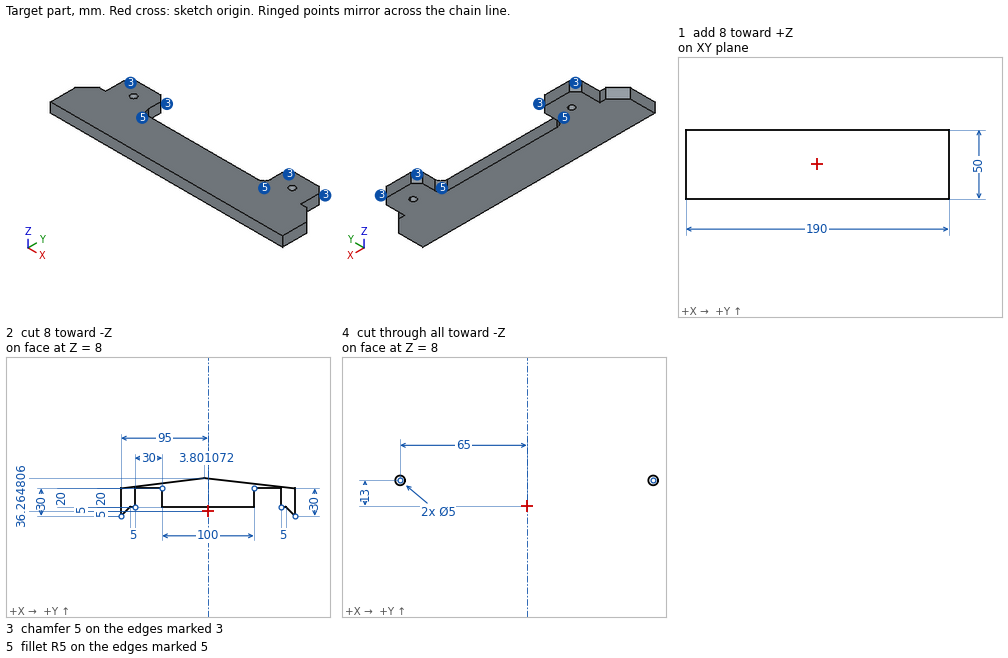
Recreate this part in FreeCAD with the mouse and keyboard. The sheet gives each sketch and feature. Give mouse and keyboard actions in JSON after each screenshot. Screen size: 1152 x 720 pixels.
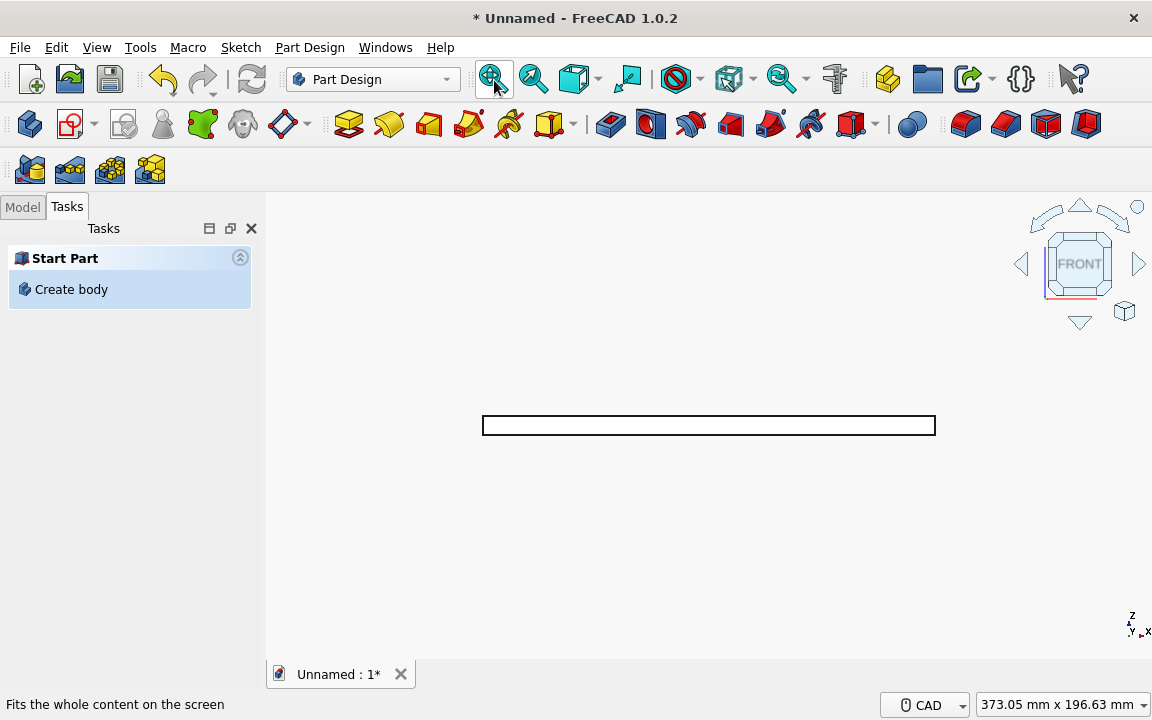
{"action": "key", "text": "3"}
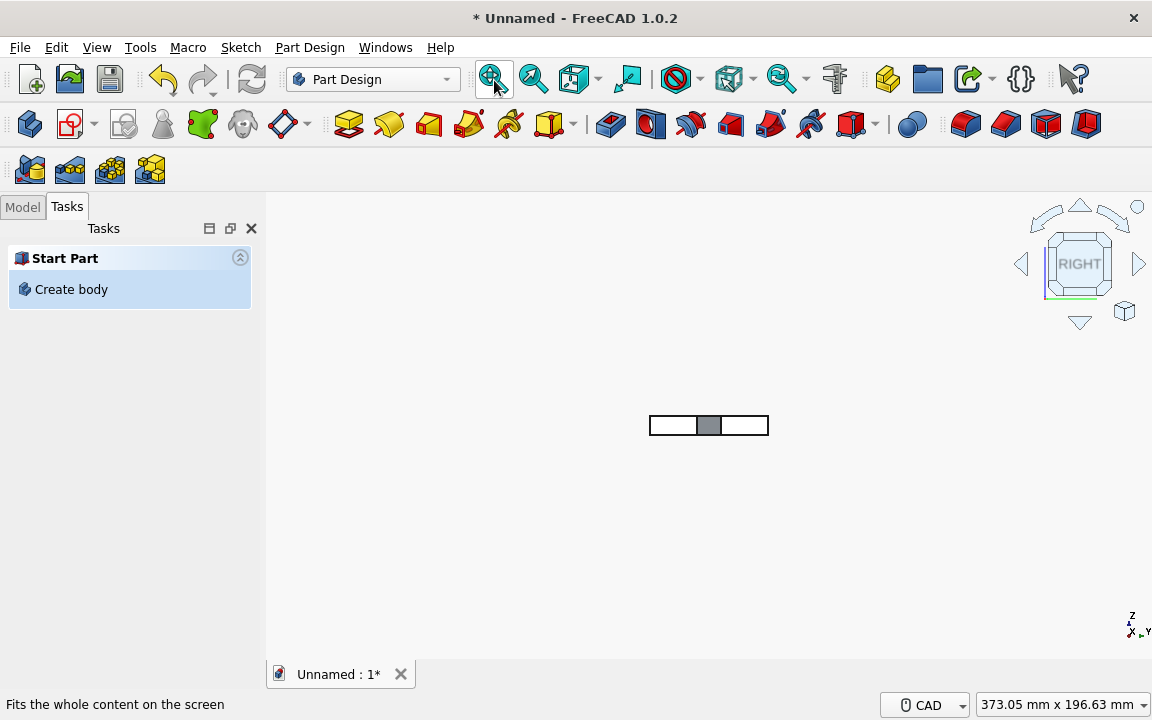
{"action": "left_click", "coordinate": [494, 80]}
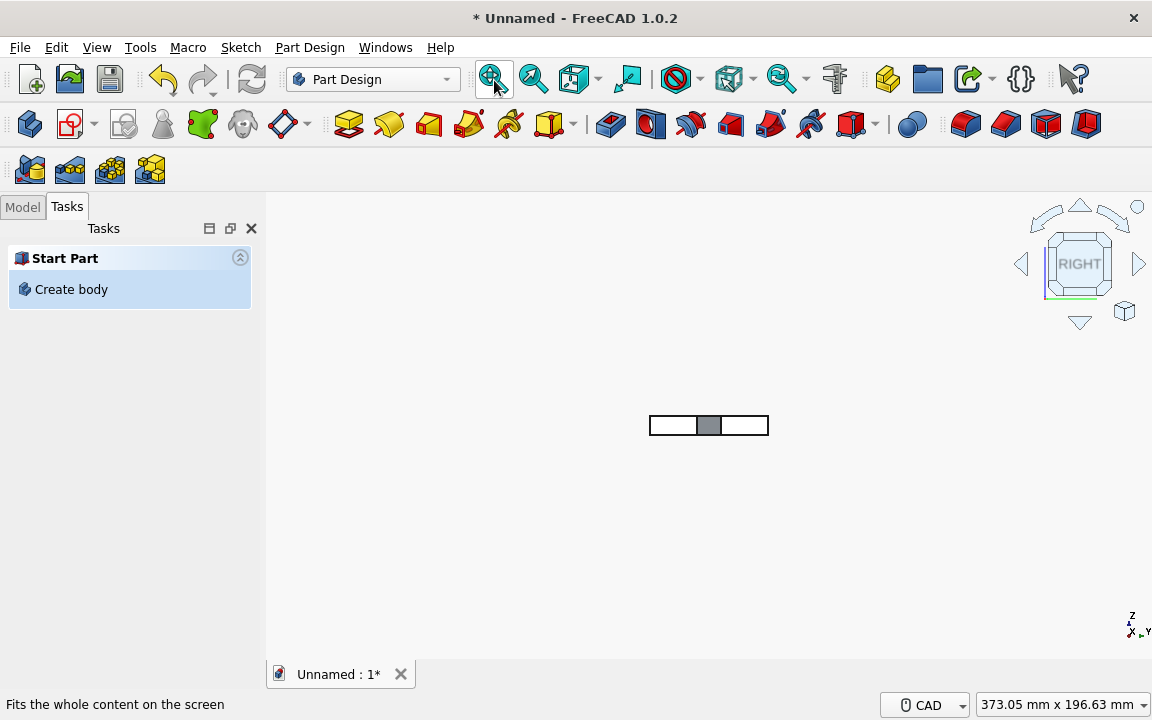
{"action": "left_click", "coordinate": [768, 424]}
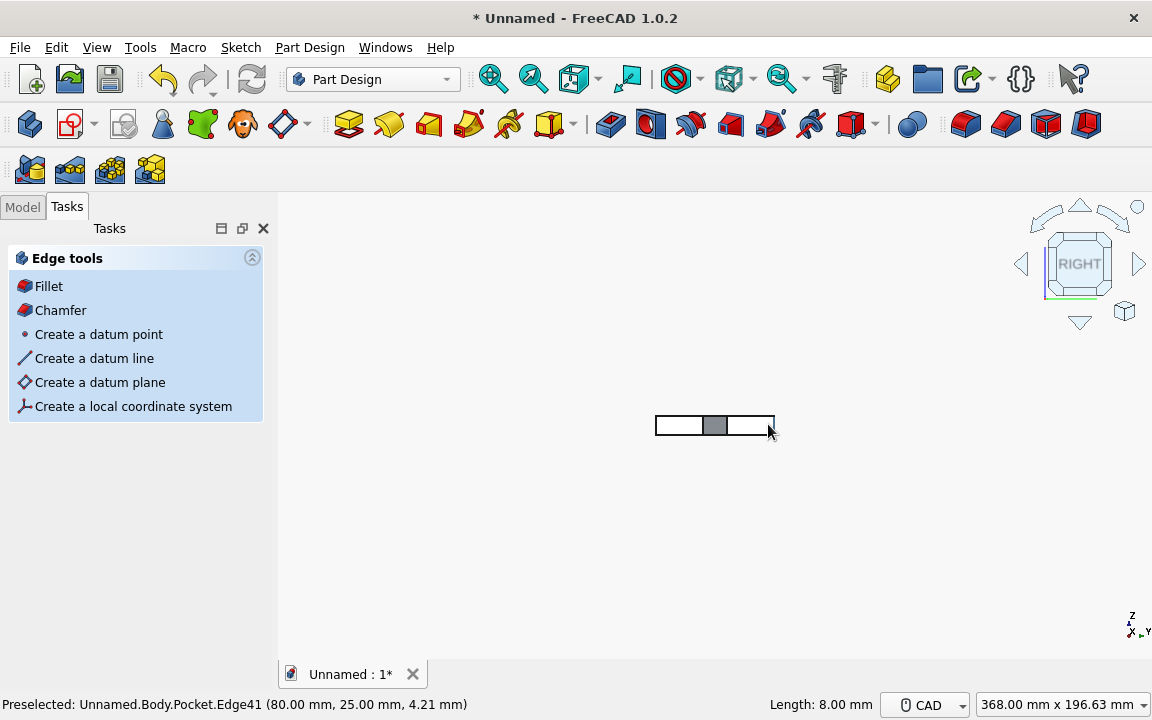
{"action": "scroll", "coordinate": [774, 424], "scroll_direction": "up", "scroll_amount": 4}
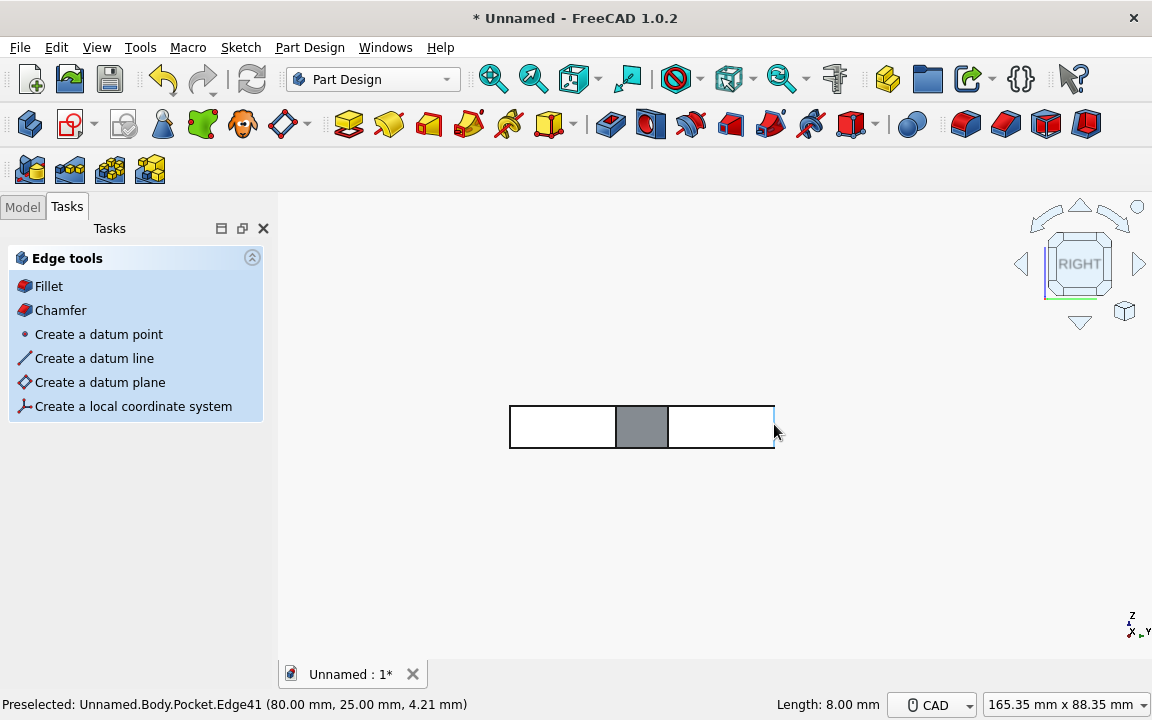
{"action": "key", "text": "v f"}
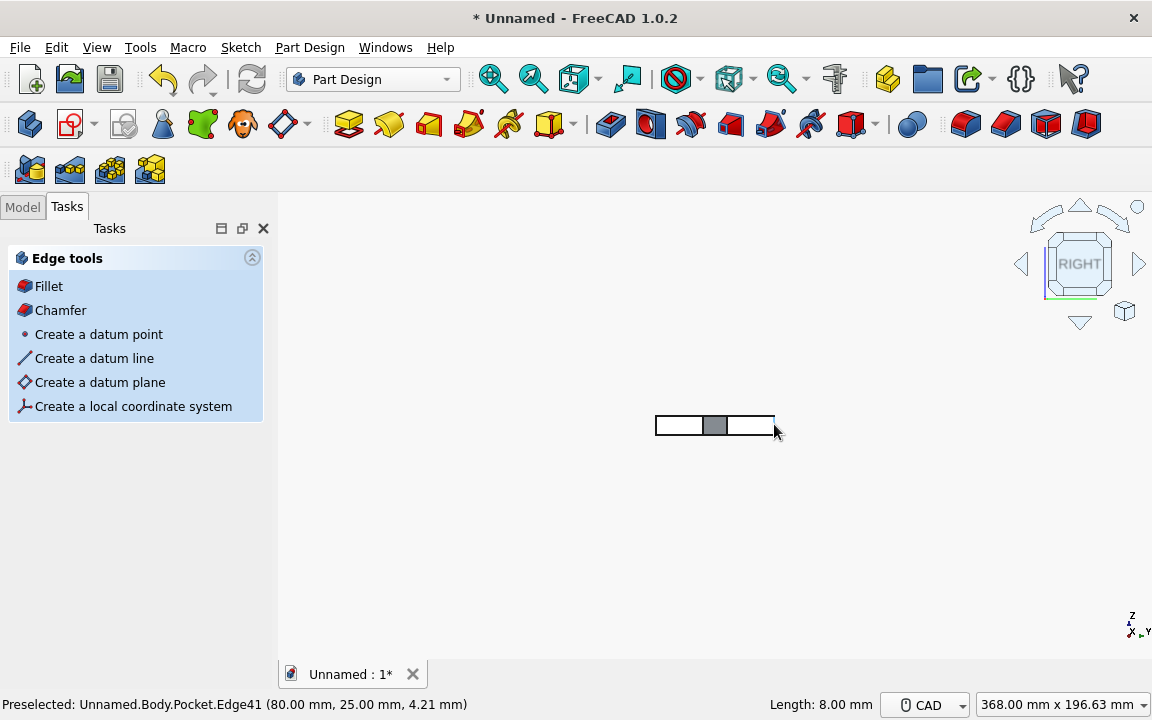
{"action": "key", "text": "5"}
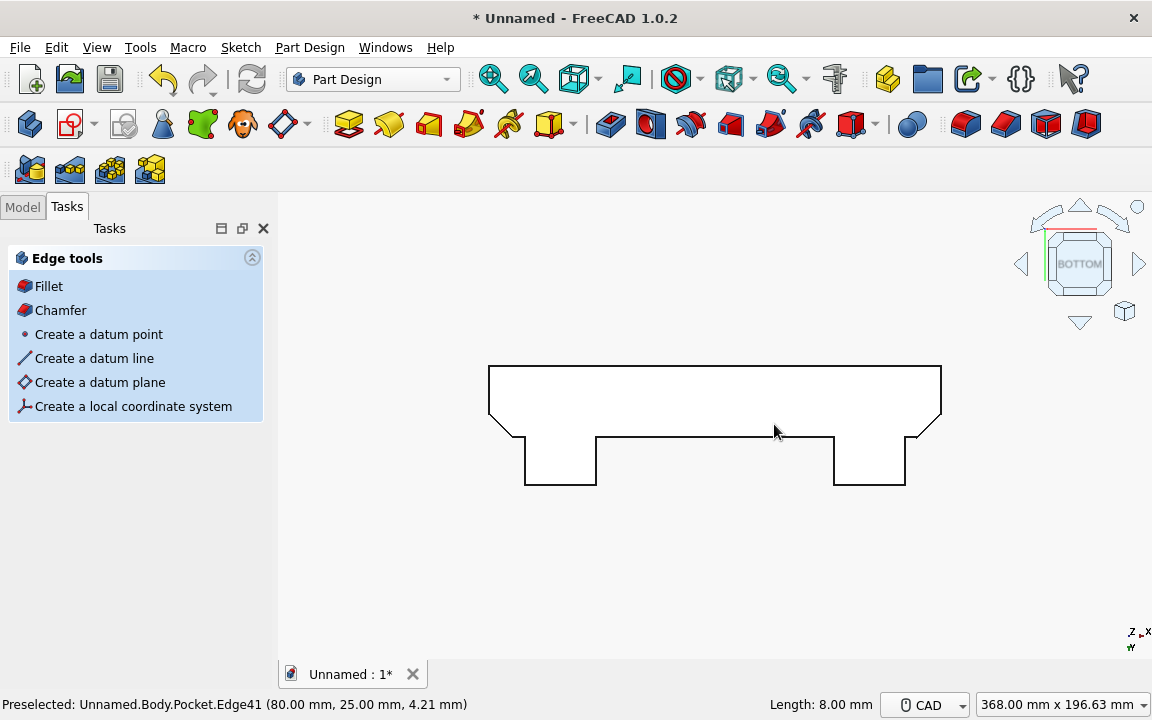
{"action": "scroll", "coordinate": [834, 484], "scroll_direction": "up", "scroll_amount": 4}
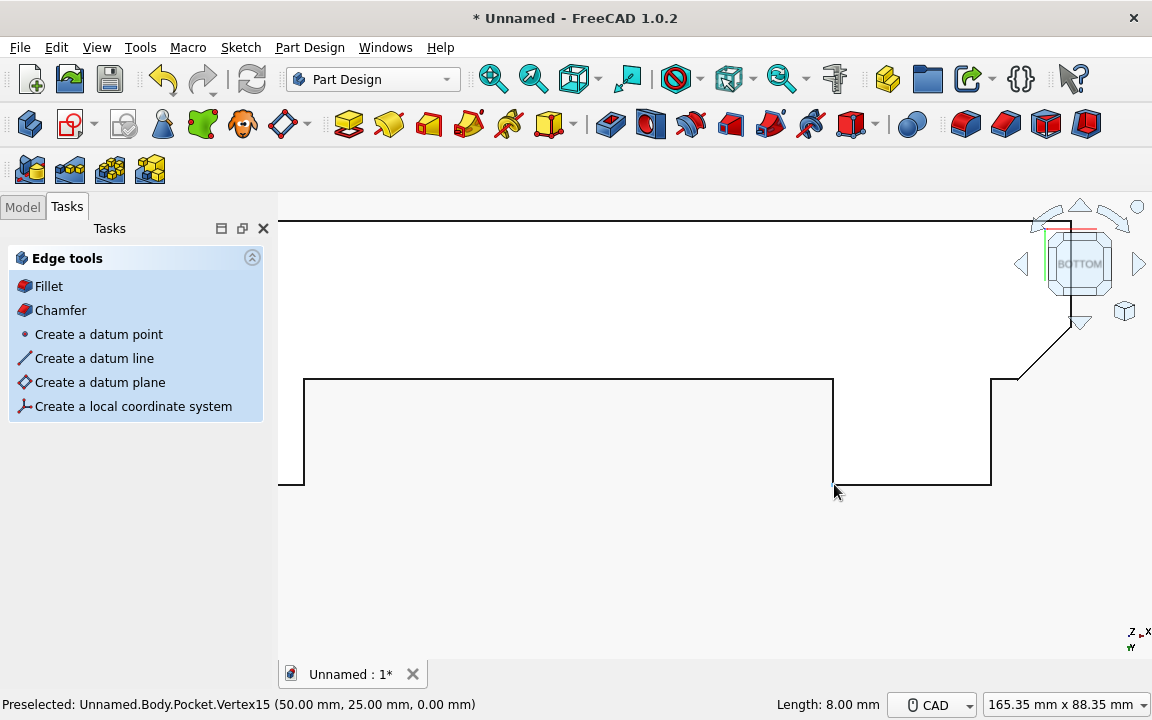
{"action": "left_click", "coordinate": [494, 80]}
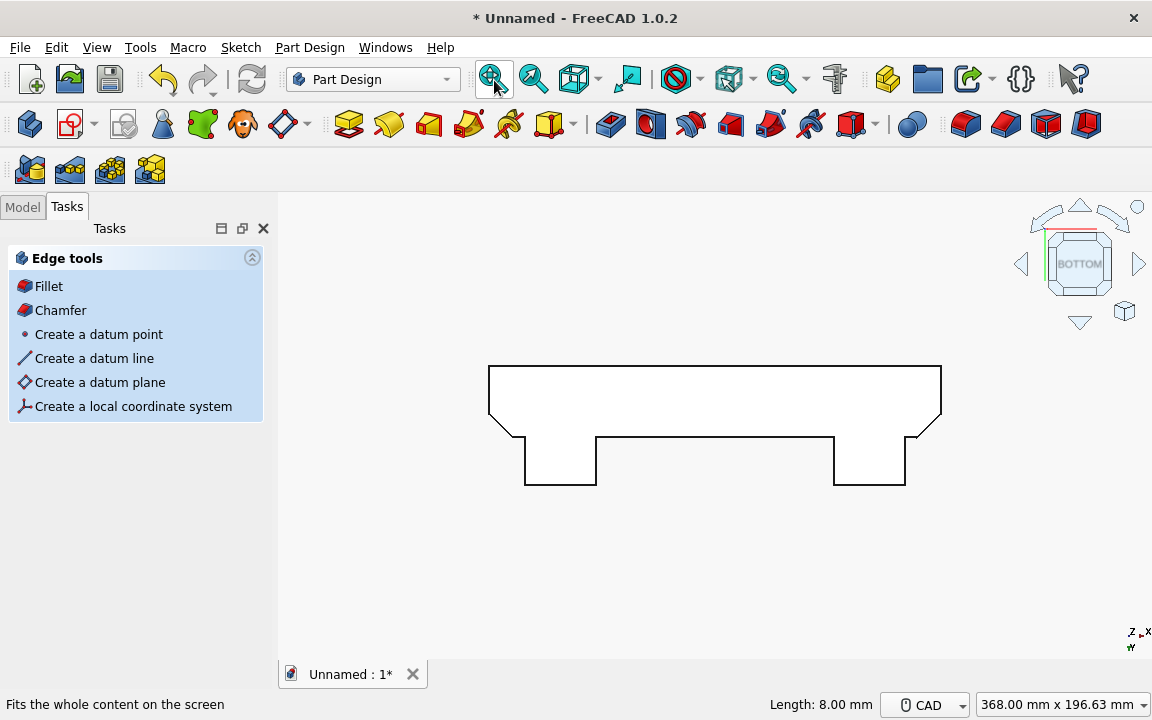
{"action": "key", "text": "4"}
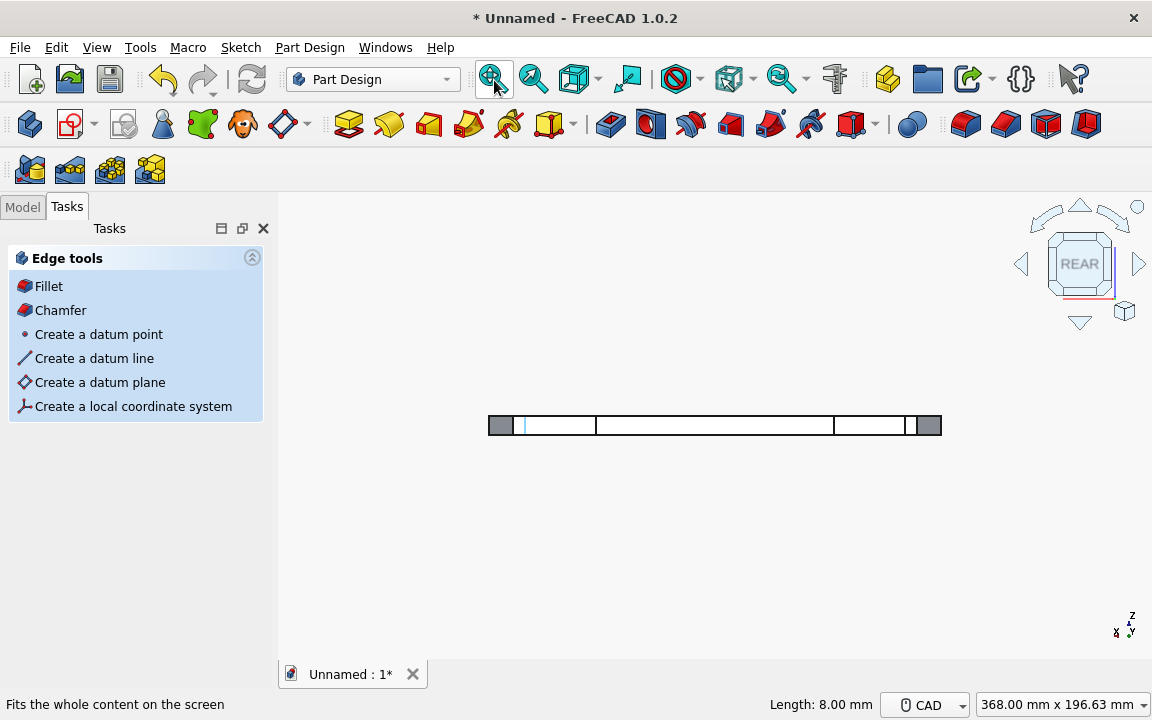
{"action": "left_click", "coordinate": [596, 424], "text": "ctrl"}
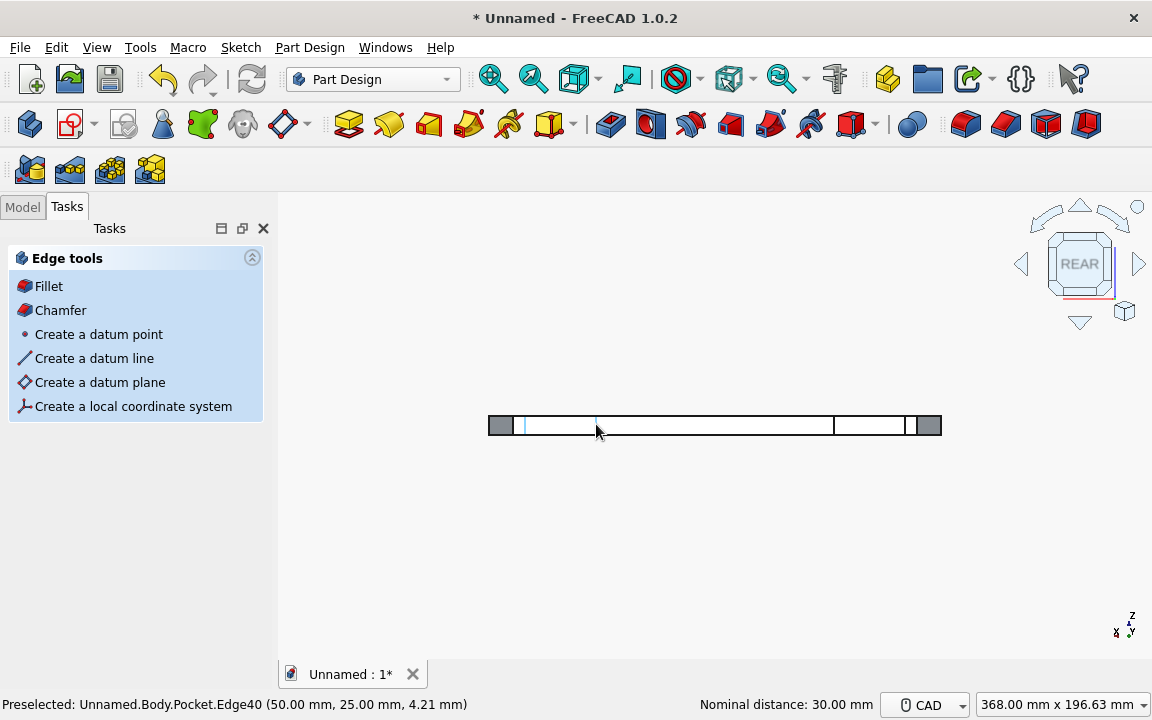
{"action": "left_click", "coordinate": [834, 424], "text": "ctrl"}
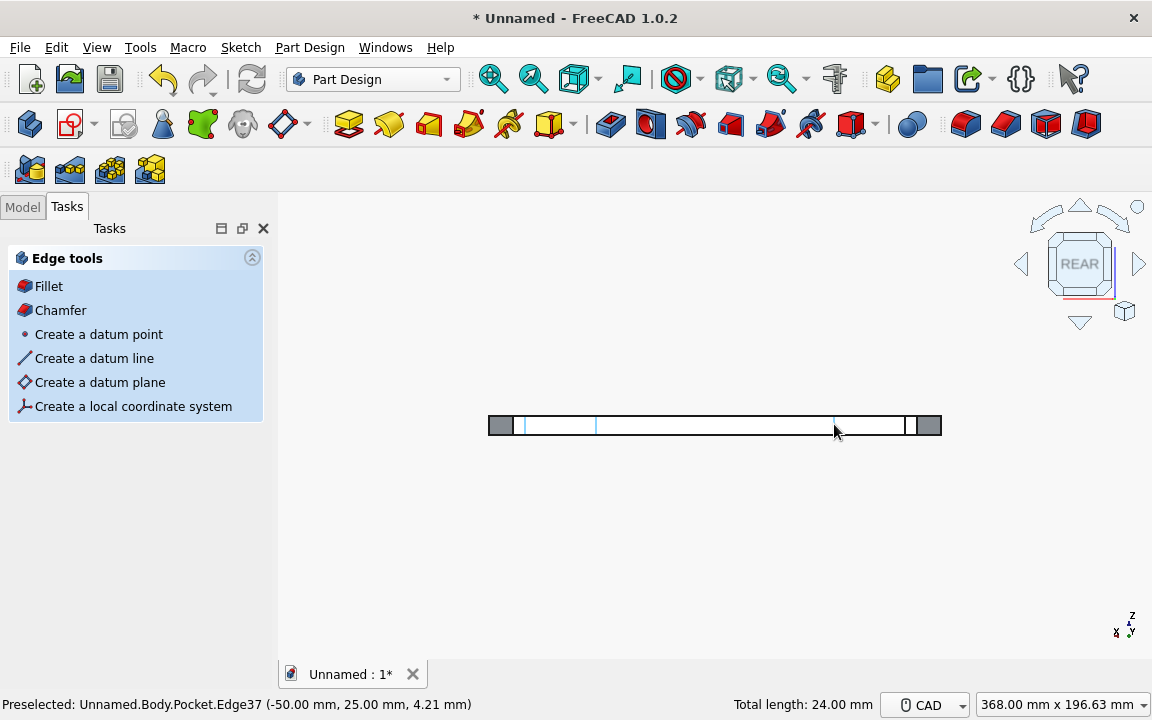
{"action": "left_click", "coordinate": [905, 424], "text": "ctrl"}